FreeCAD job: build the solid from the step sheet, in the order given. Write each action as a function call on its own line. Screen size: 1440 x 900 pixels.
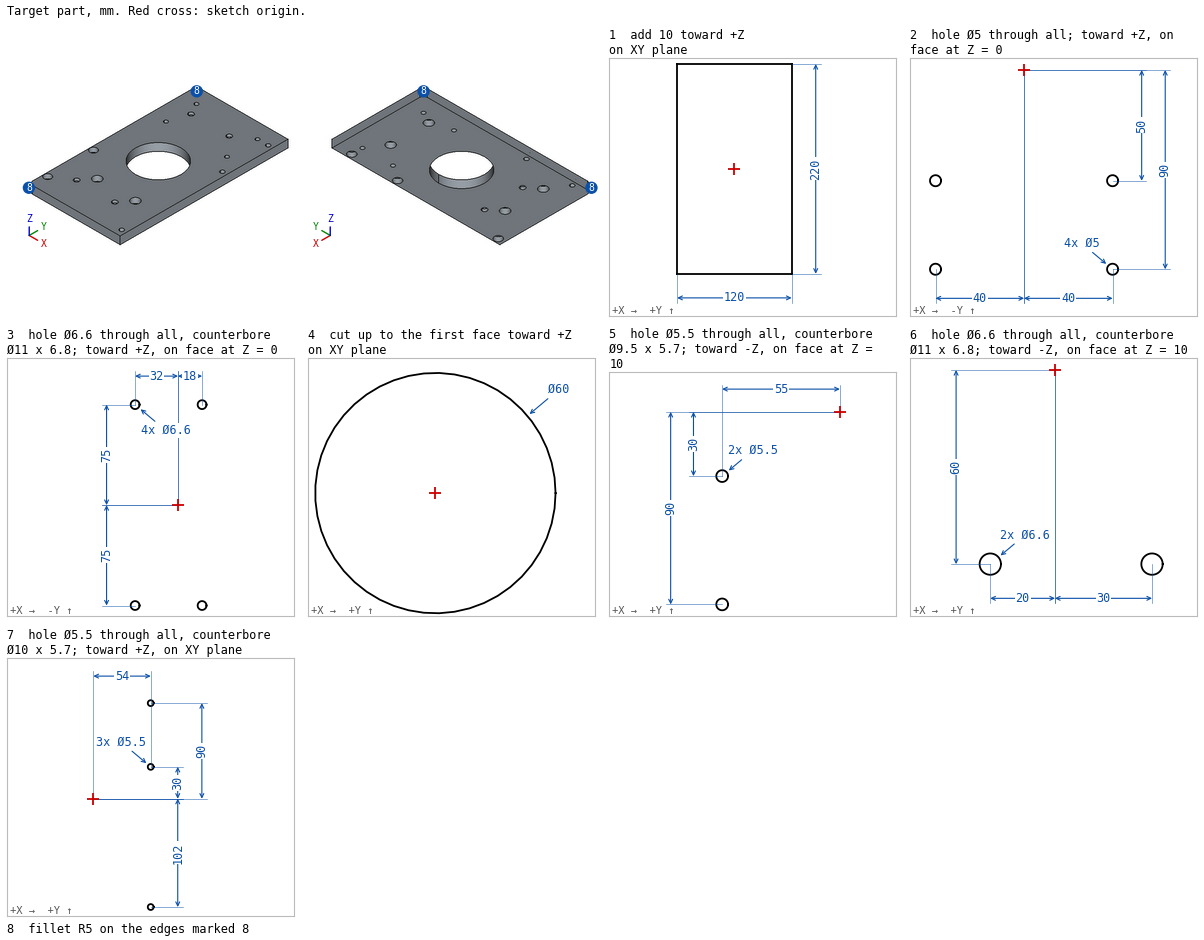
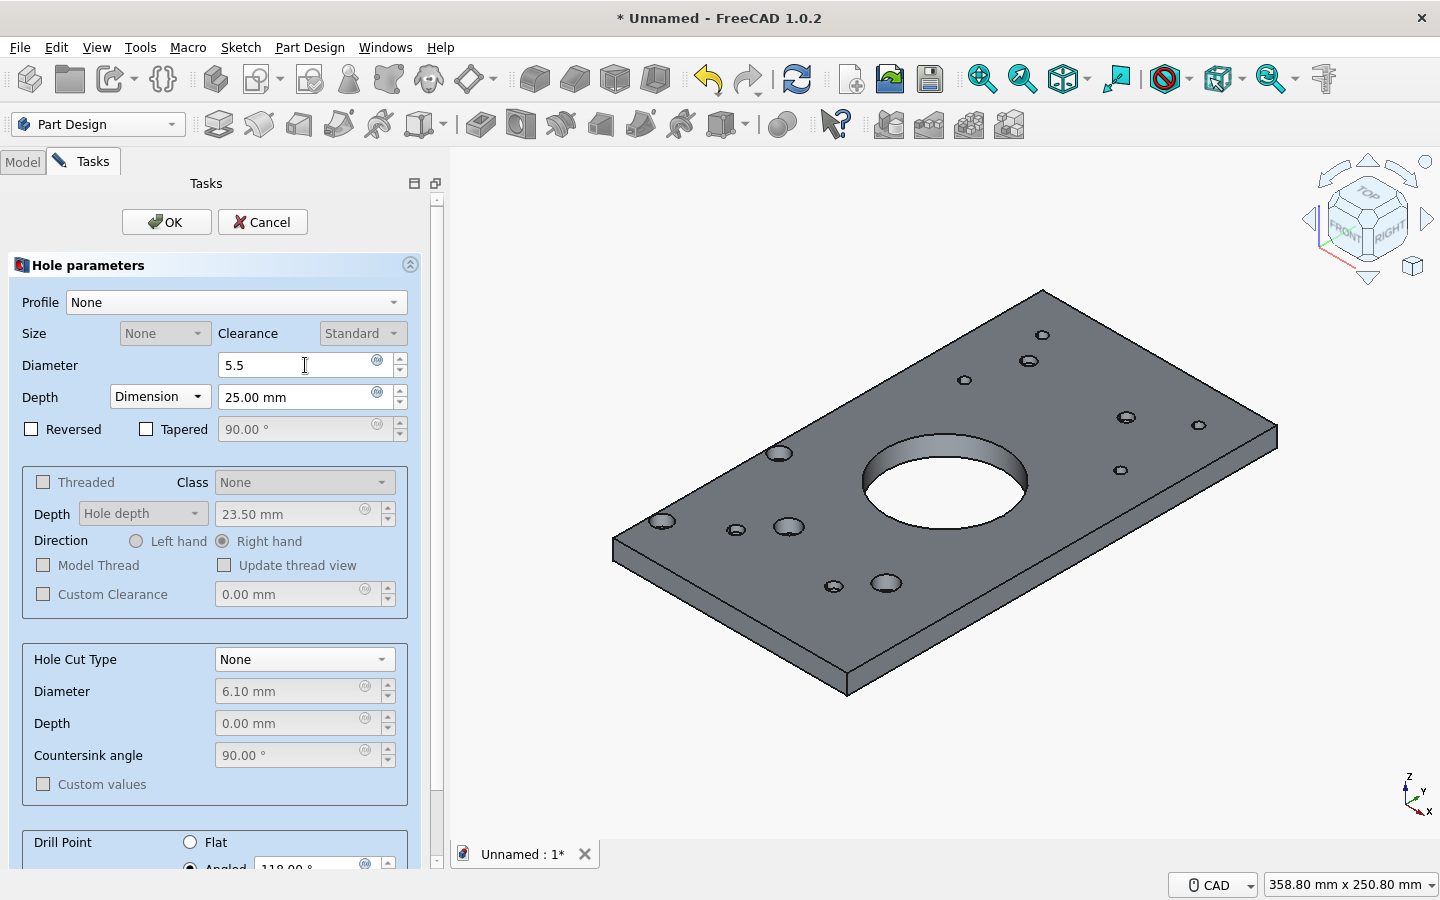
click(161, 396)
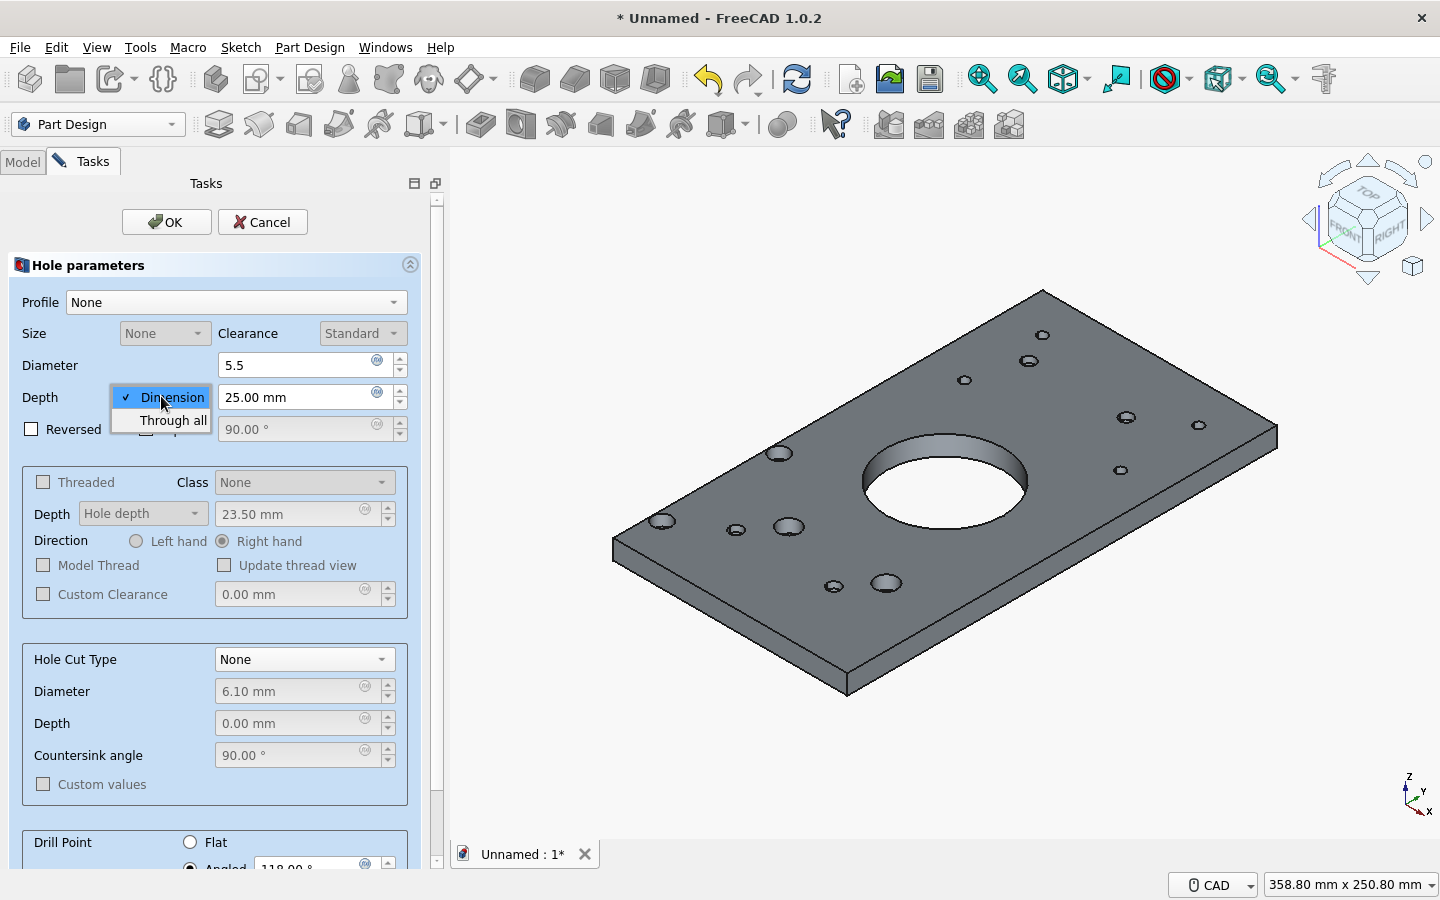
click(160, 420)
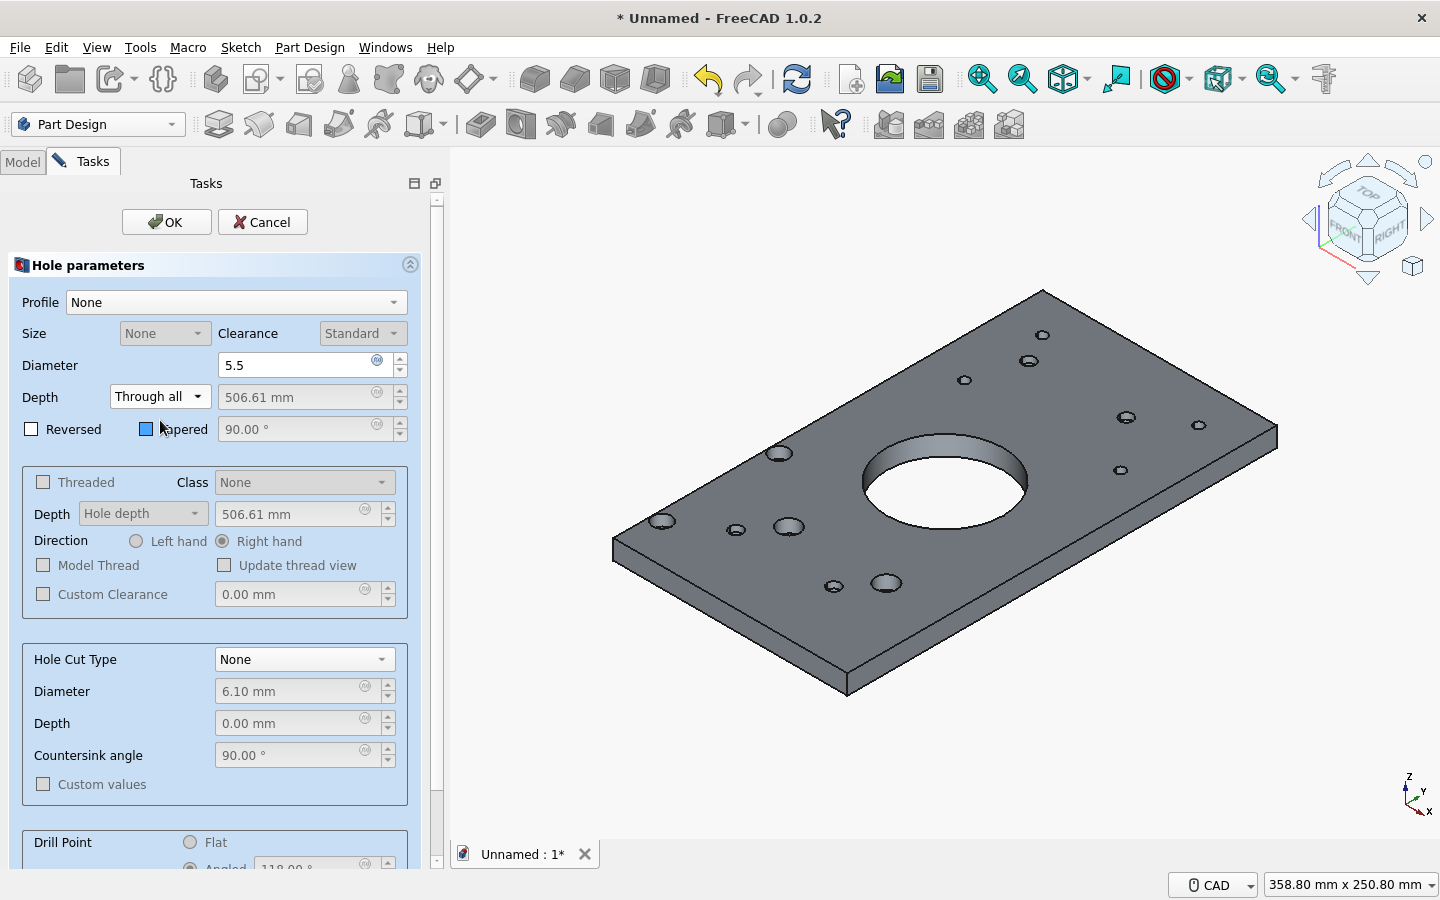
click(30, 429)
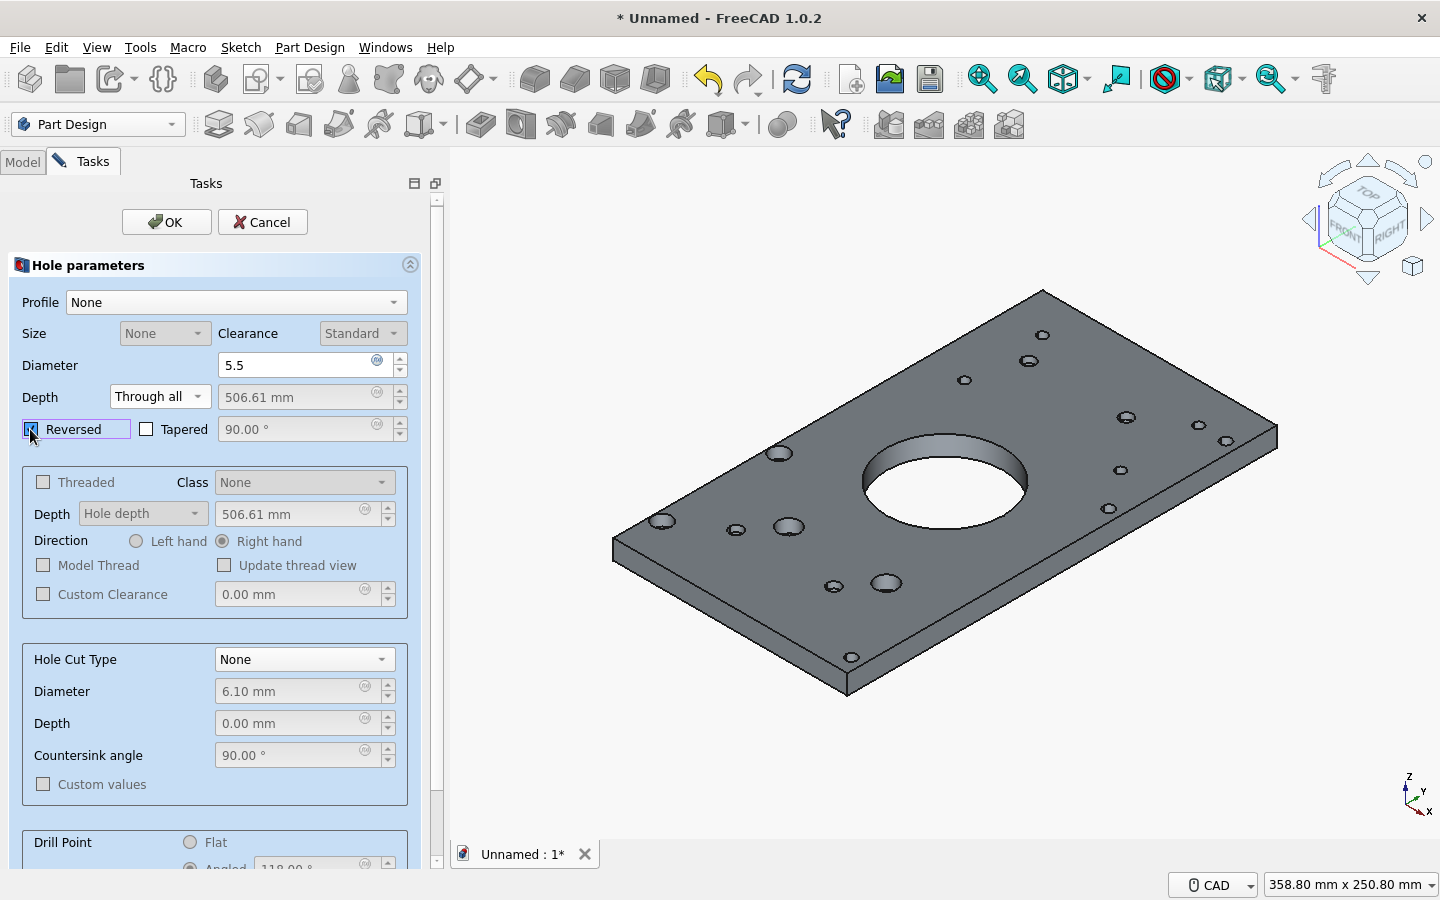
click(306, 660)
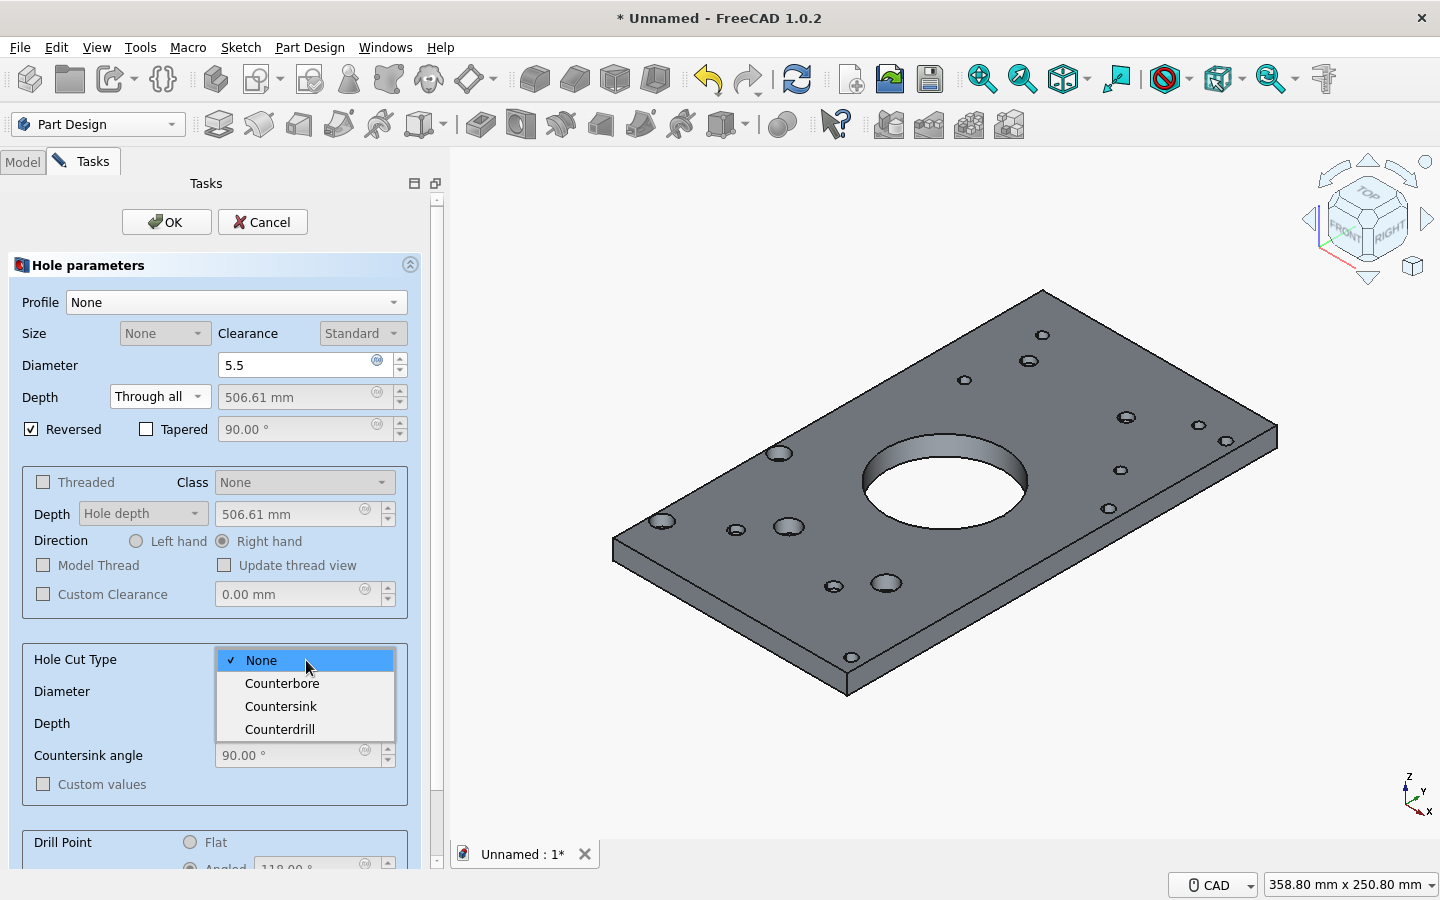
click(304, 684)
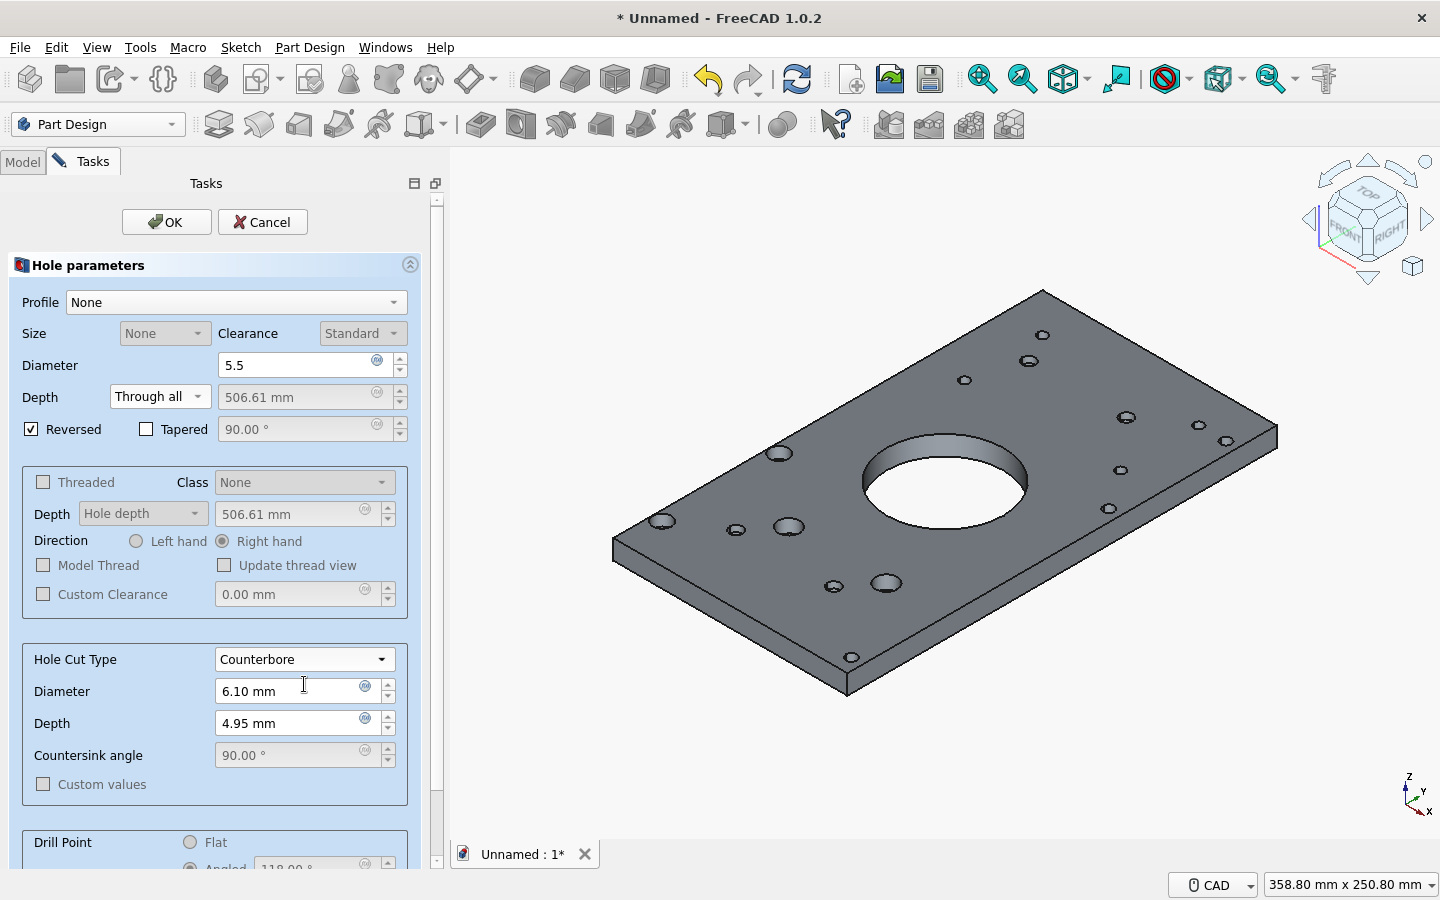
triple_click(298, 691)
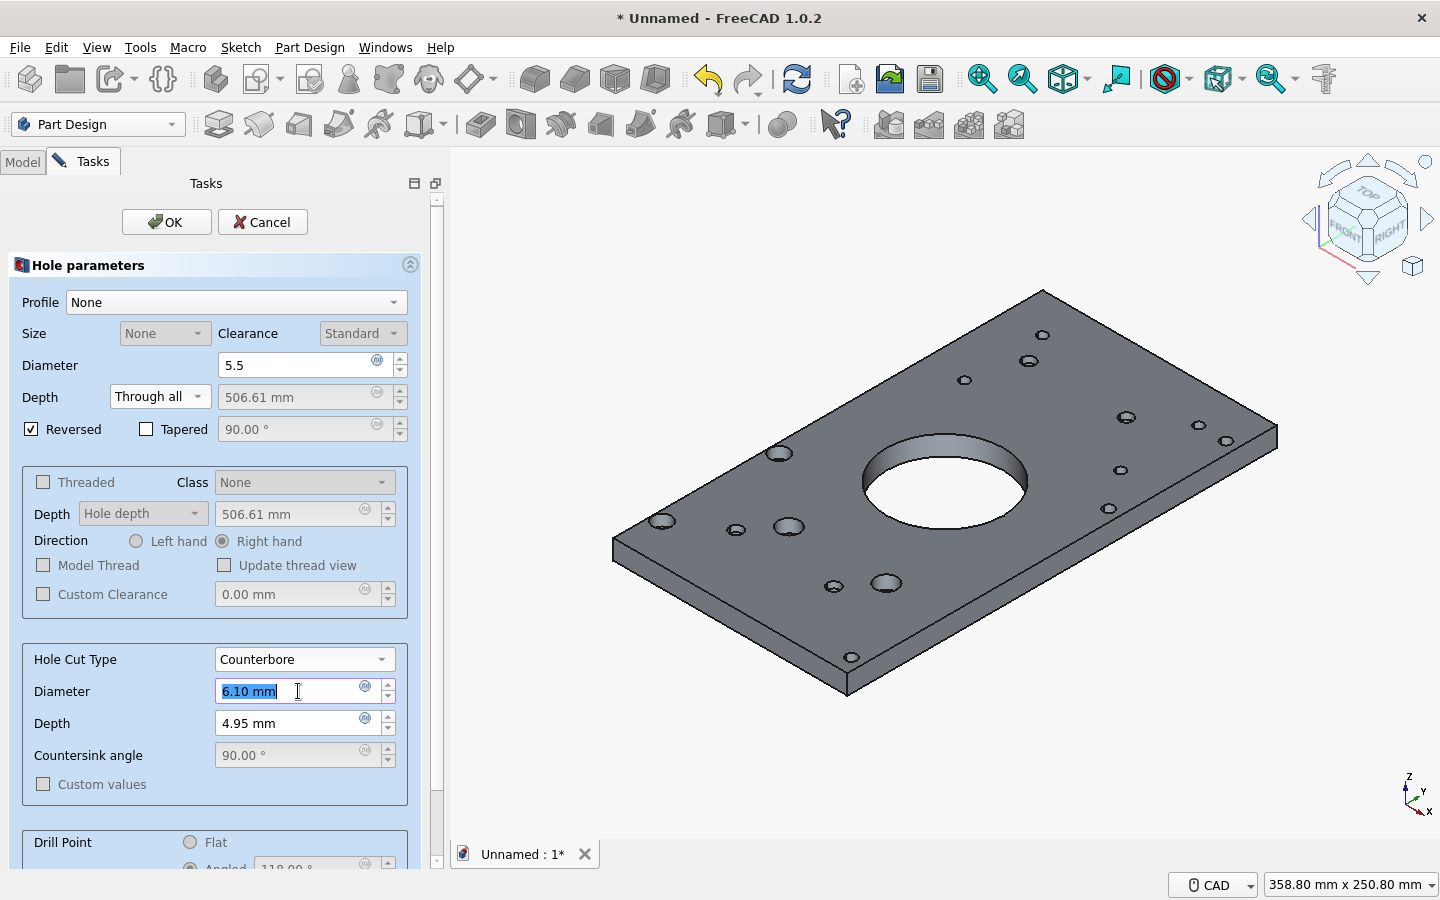
text(10)
key(Tab)